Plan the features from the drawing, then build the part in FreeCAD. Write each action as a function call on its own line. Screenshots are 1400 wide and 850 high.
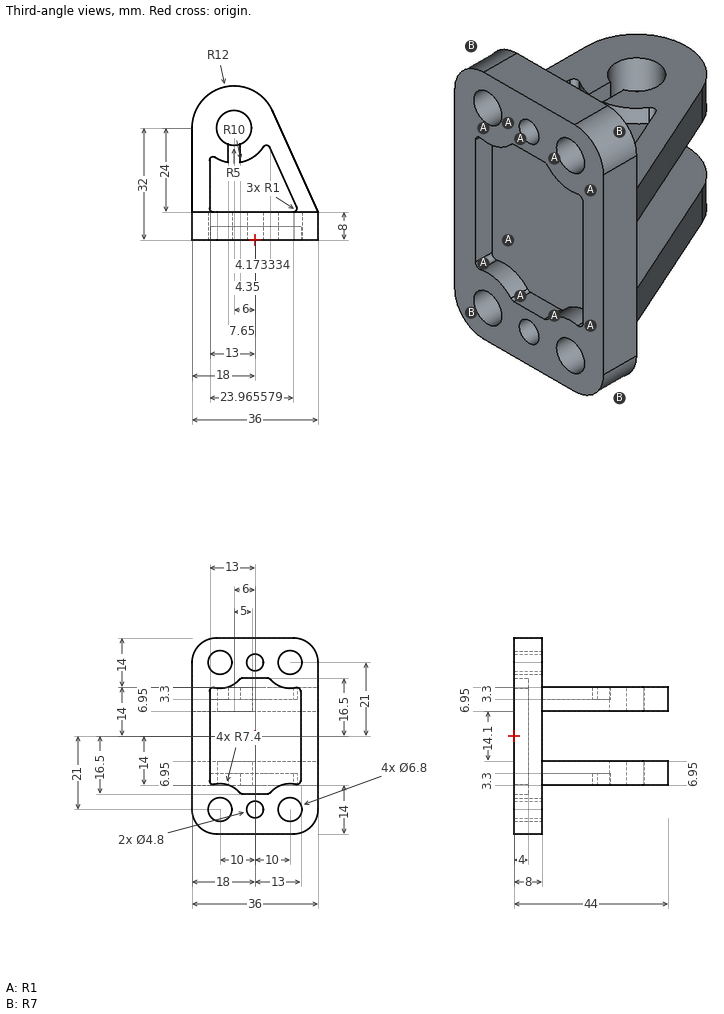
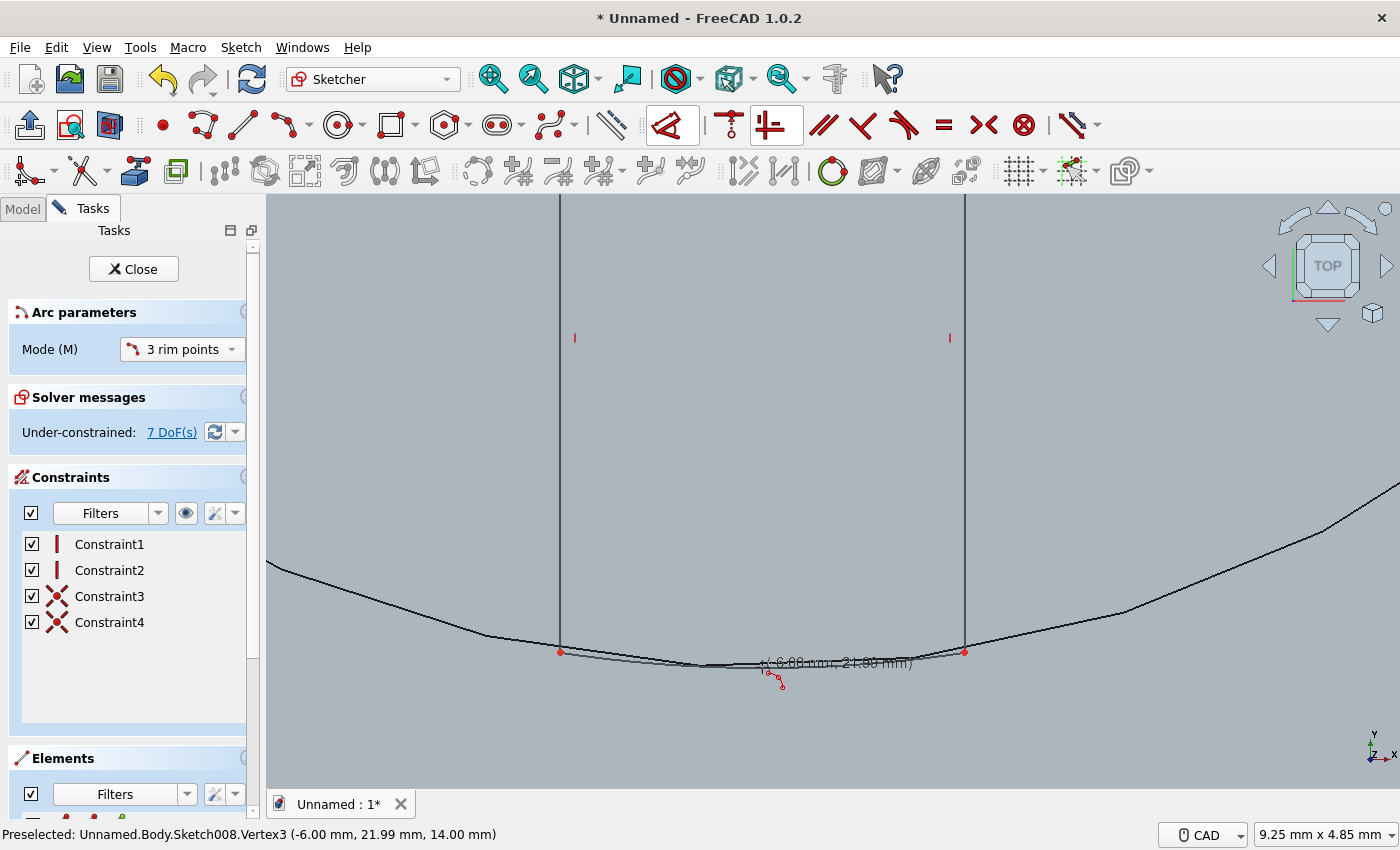
scroll(768, 671, down, 3)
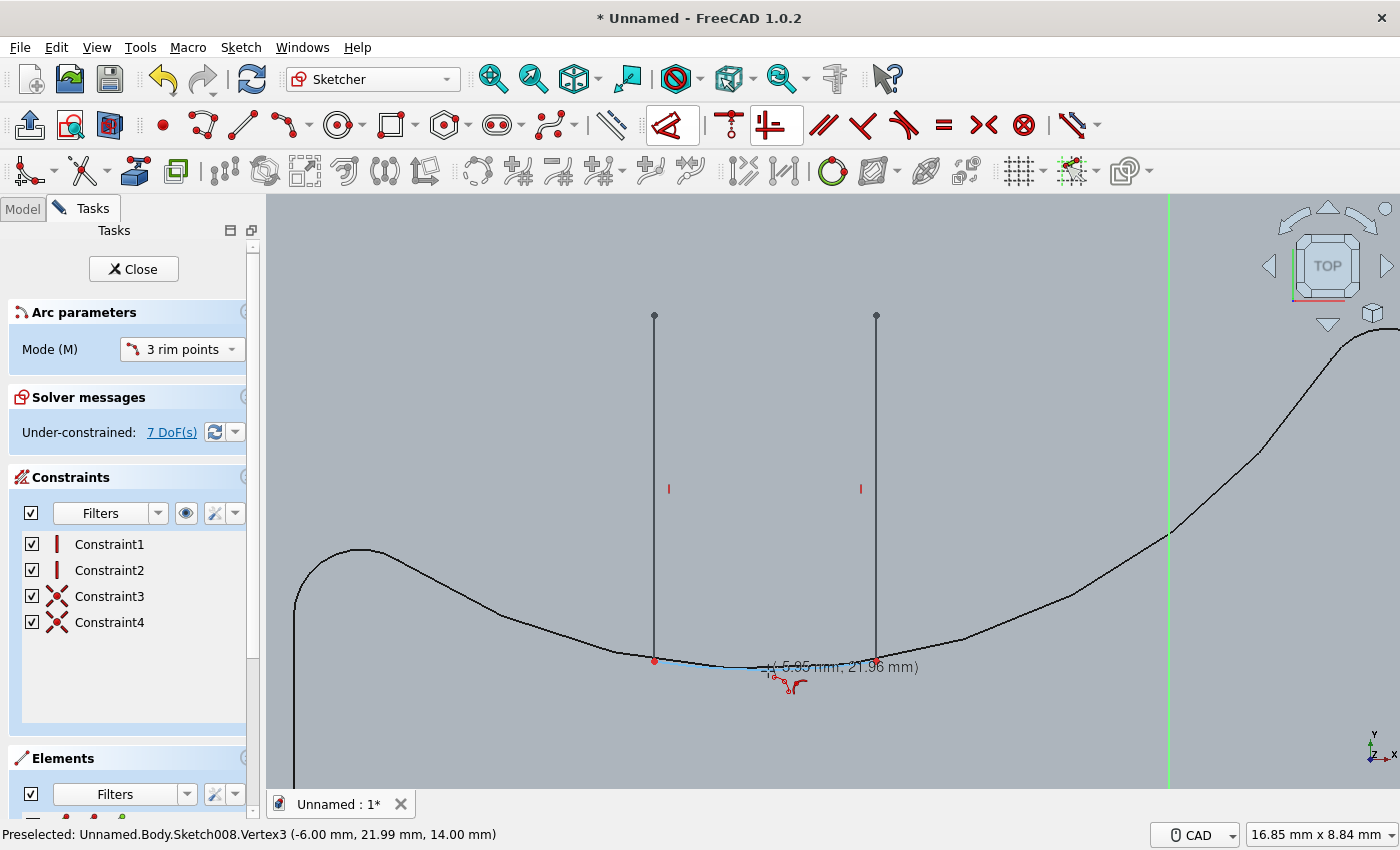
click(876, 315)
click(654, 315)
click(765, 333)
key(Escape)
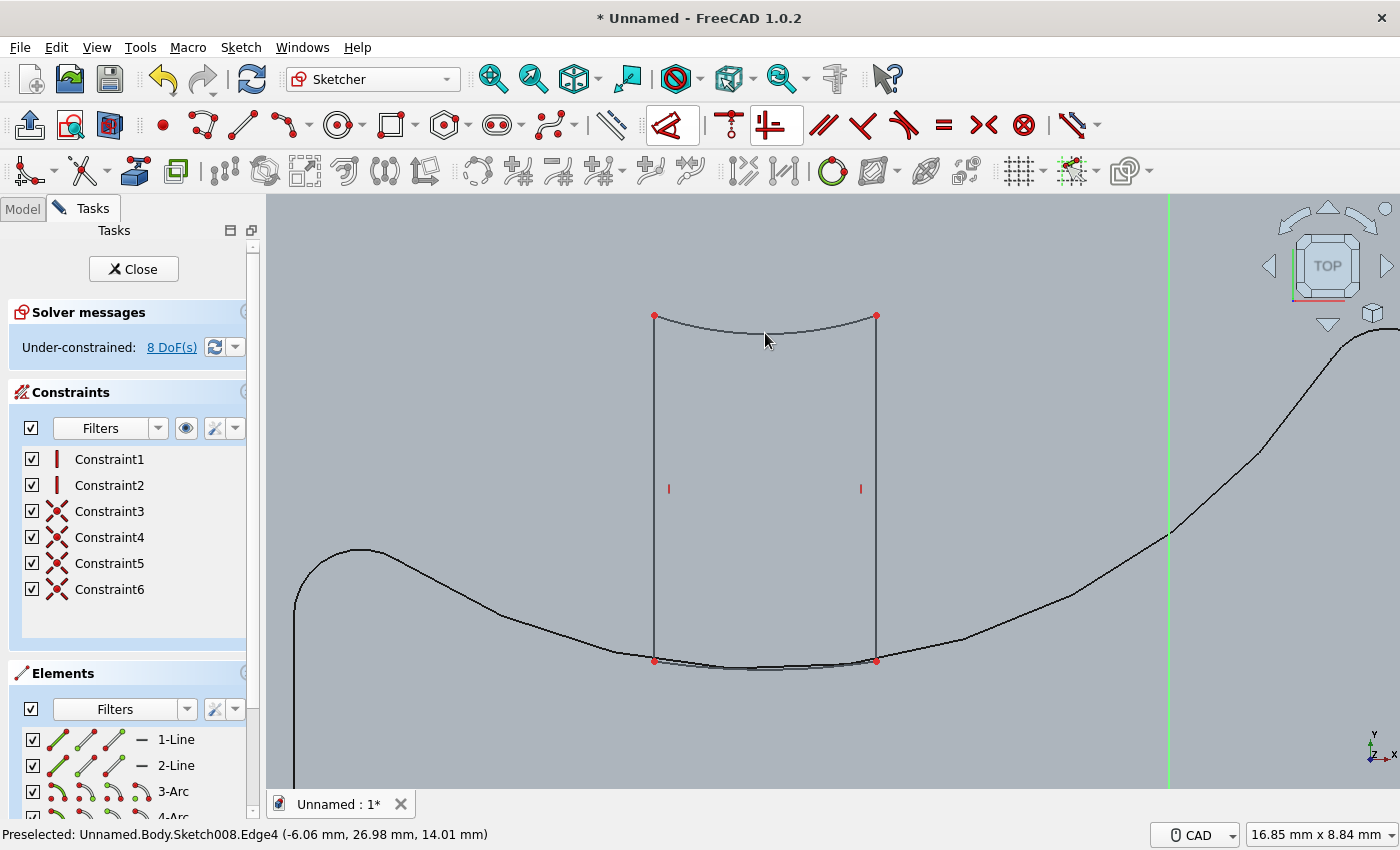
click(721, 668)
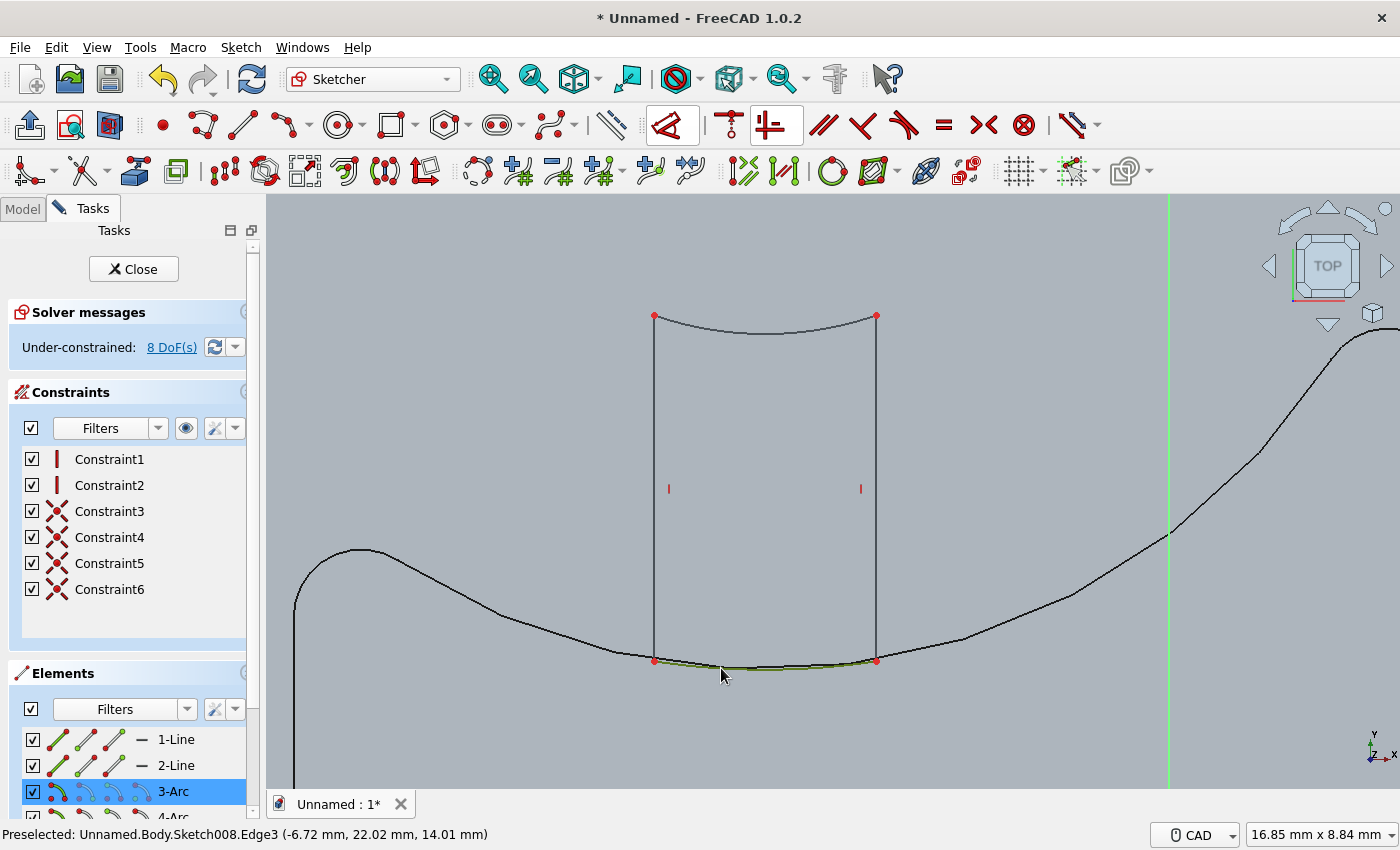
click(720, 331)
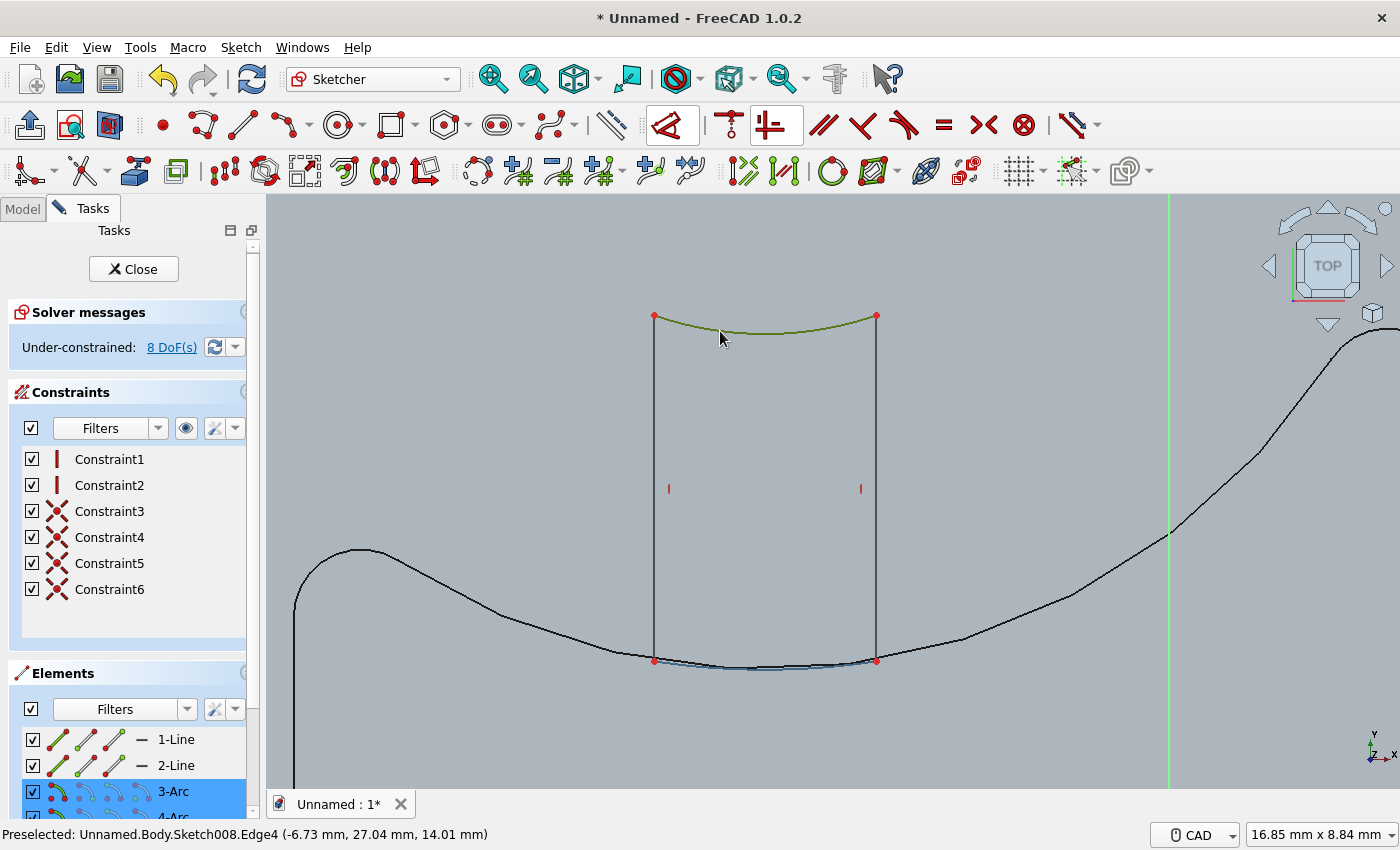
click(730, 126)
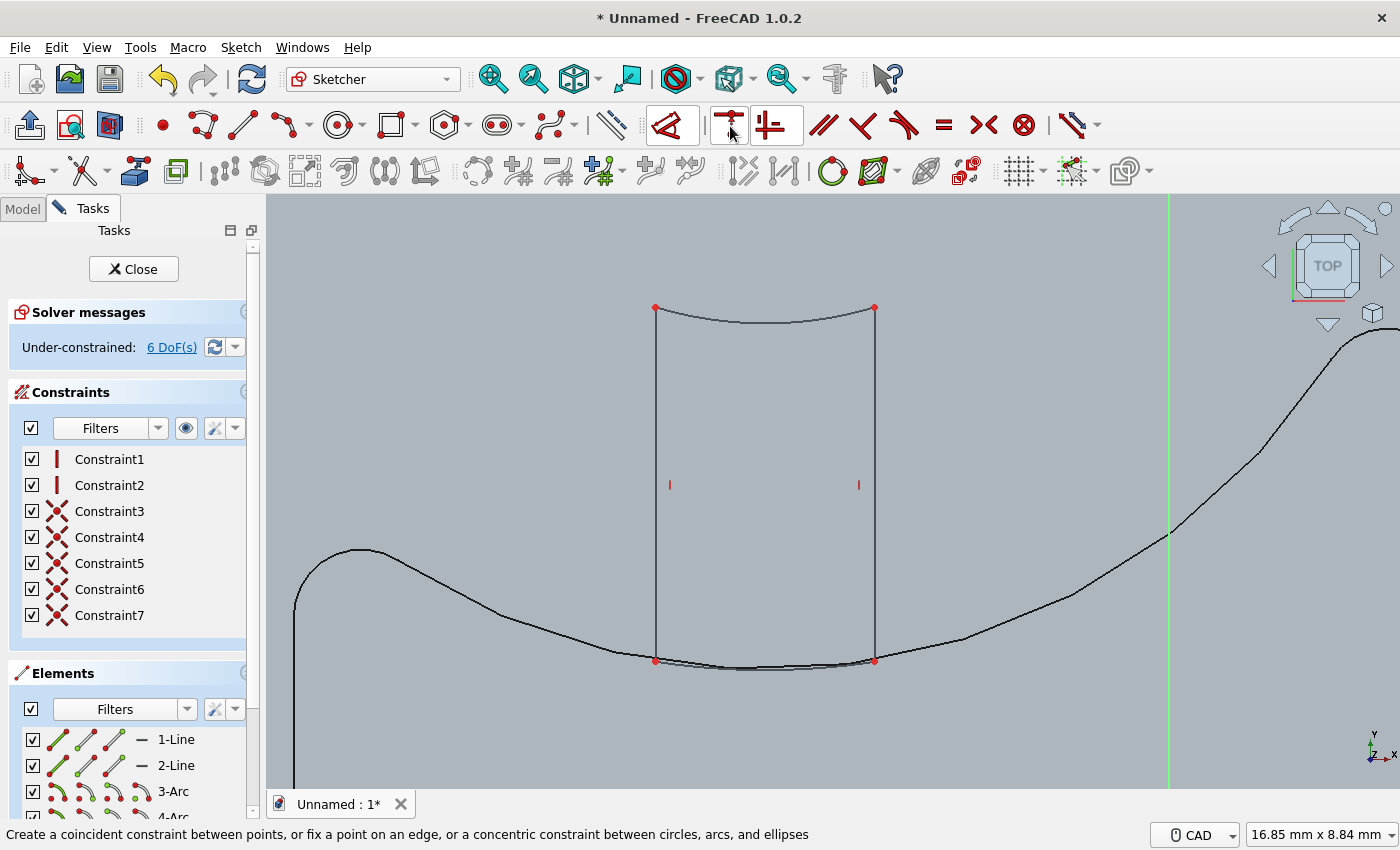
click(721, 669)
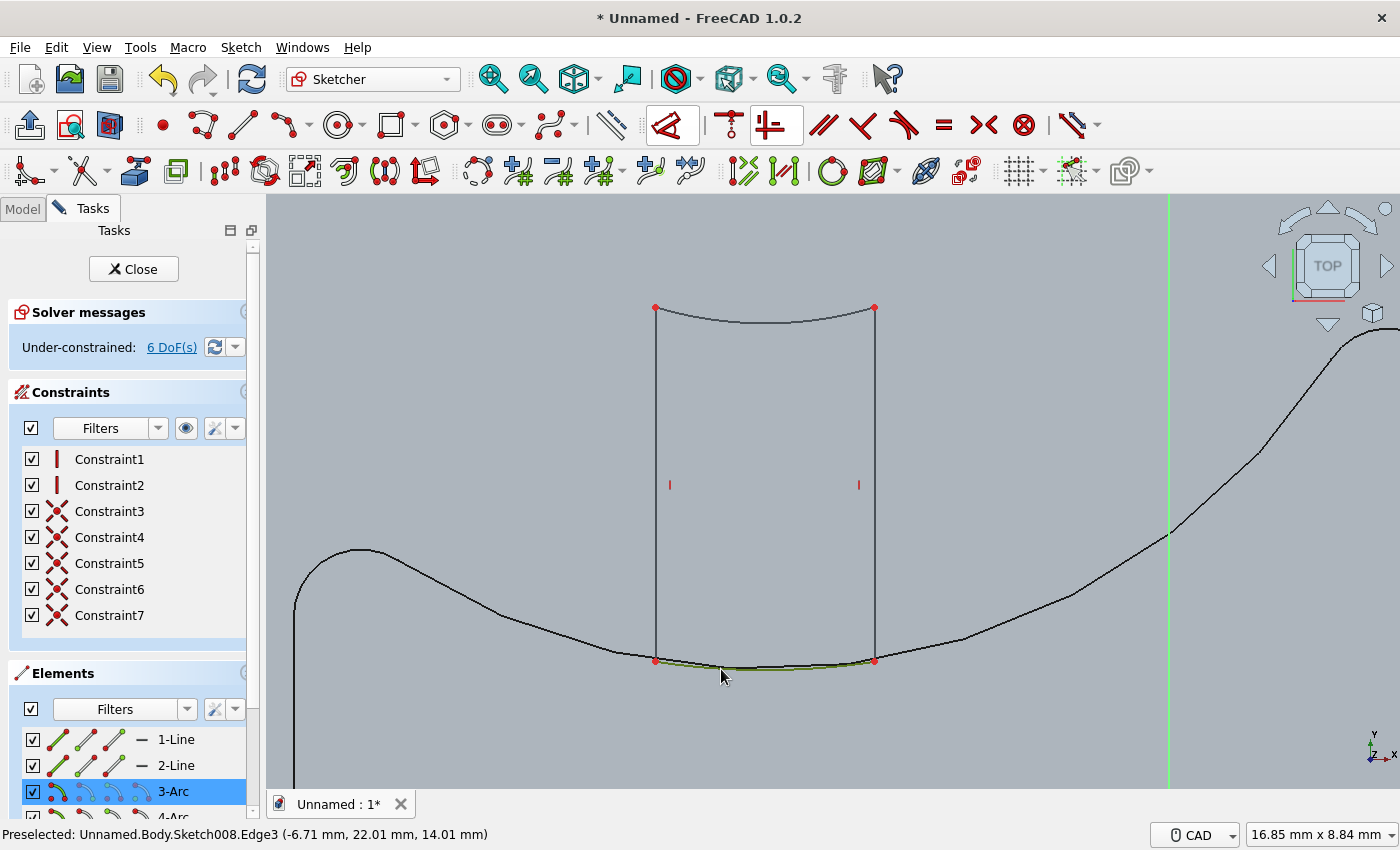
click(694, 126)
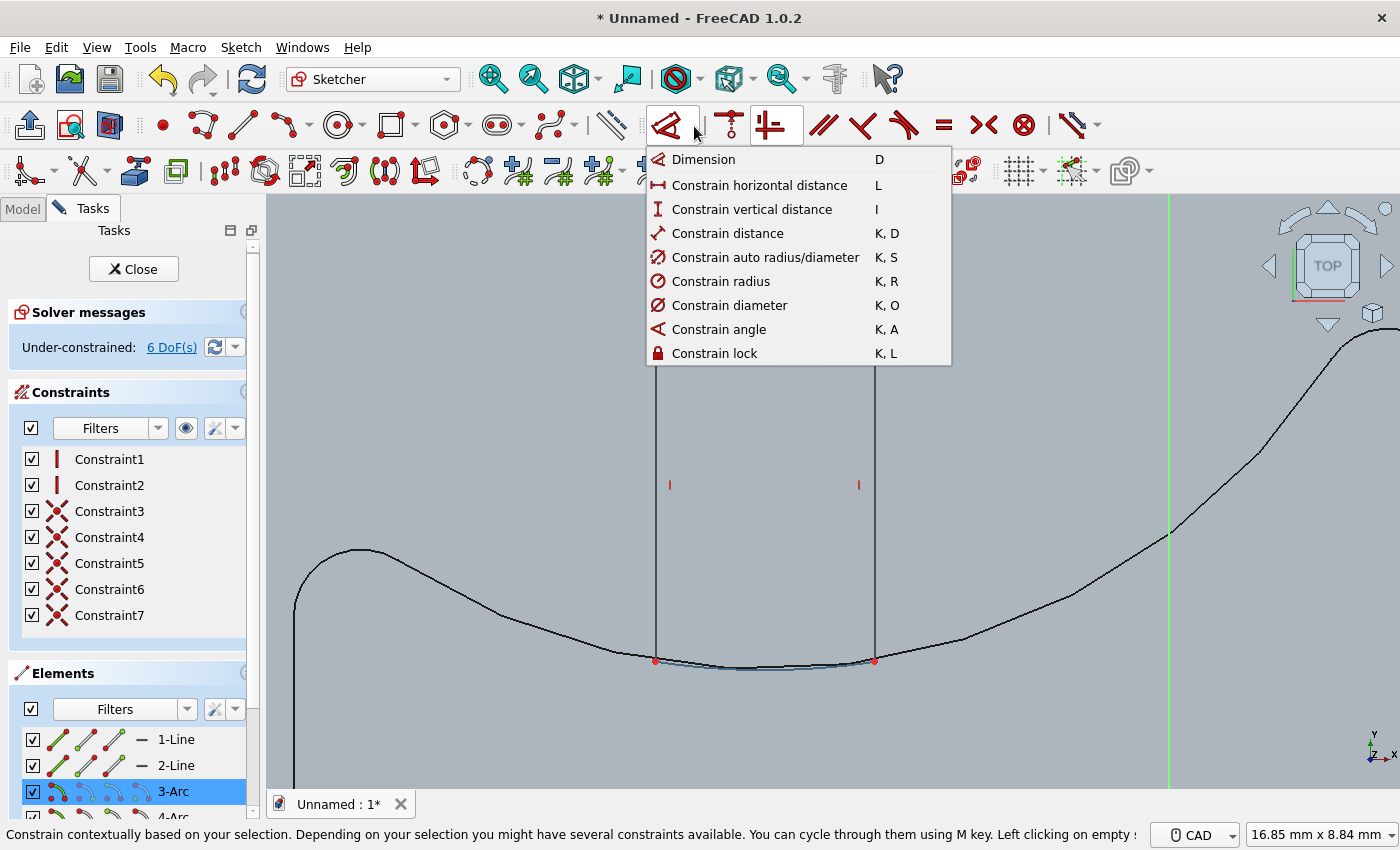
click(799, 281)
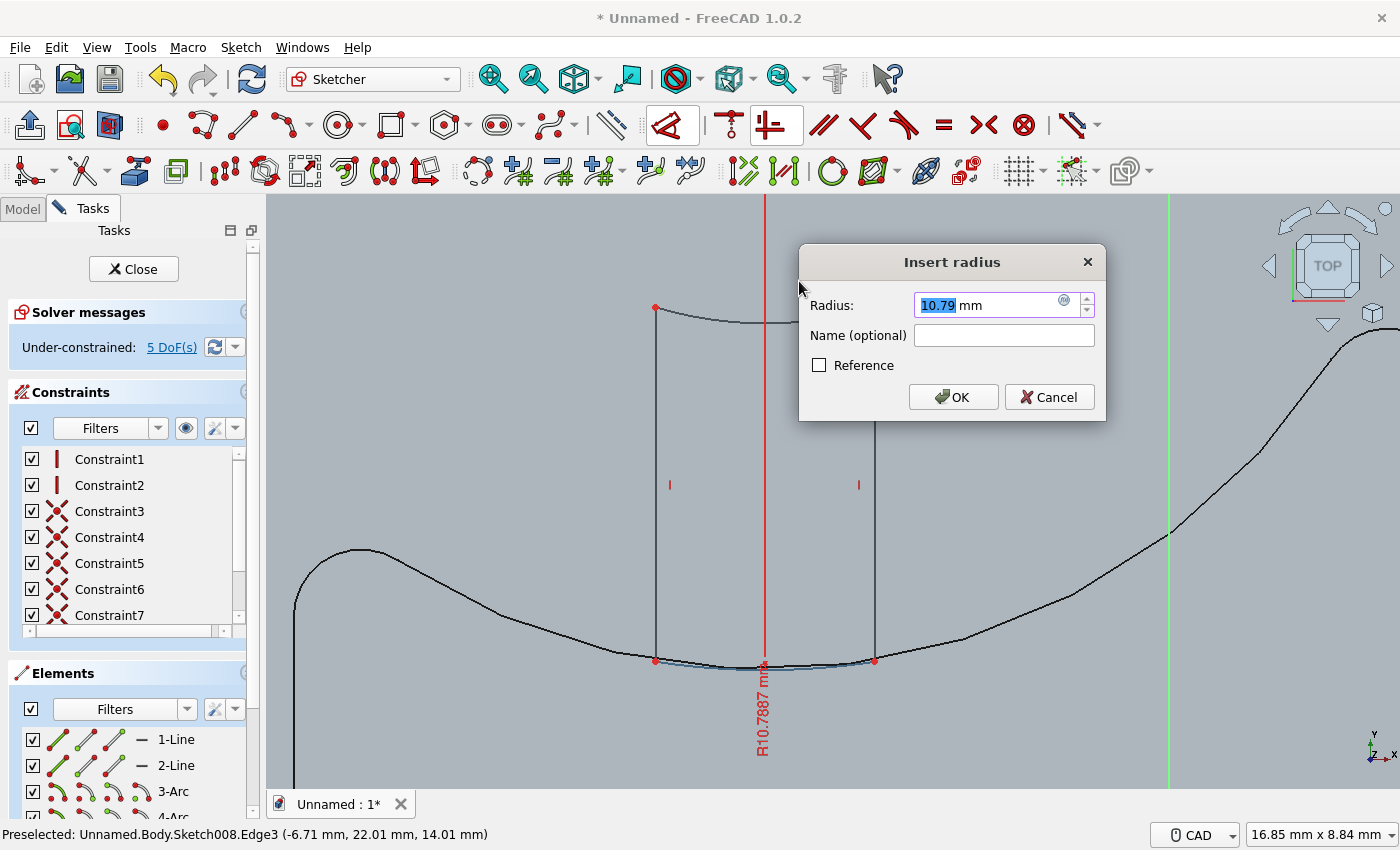
text(10)
key(Return)